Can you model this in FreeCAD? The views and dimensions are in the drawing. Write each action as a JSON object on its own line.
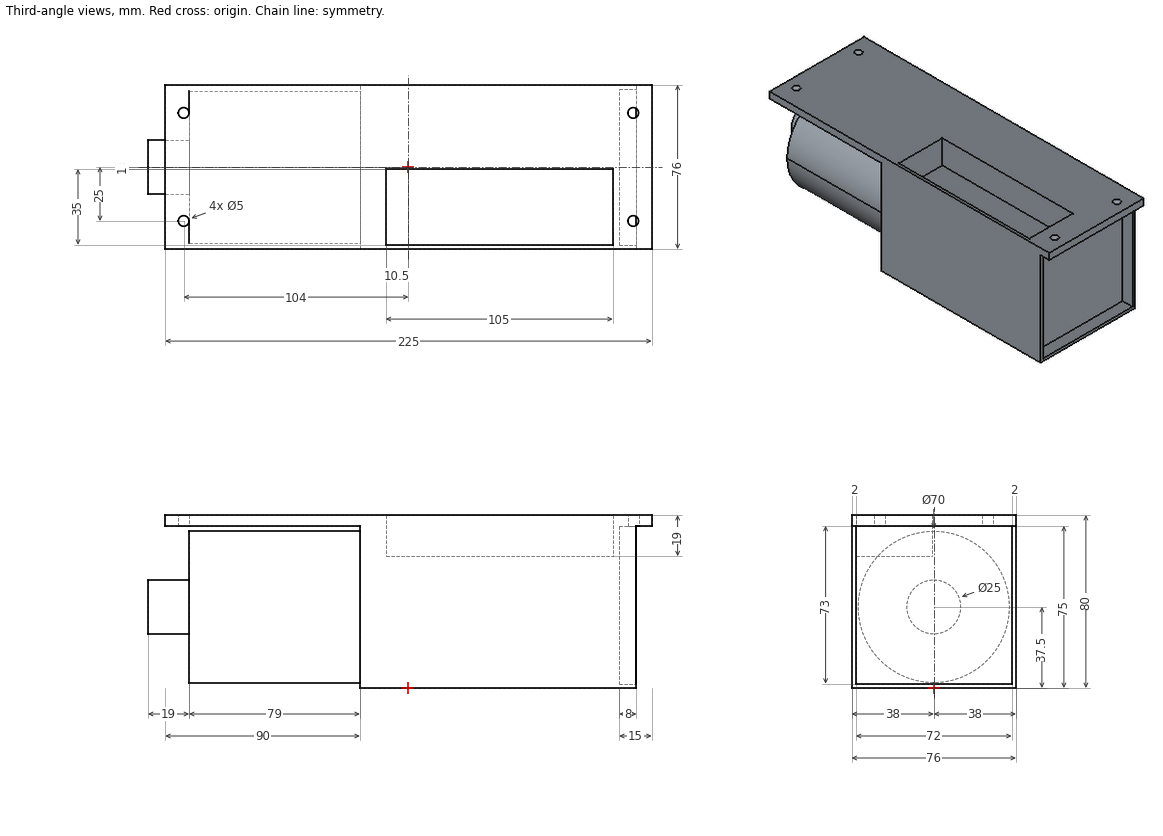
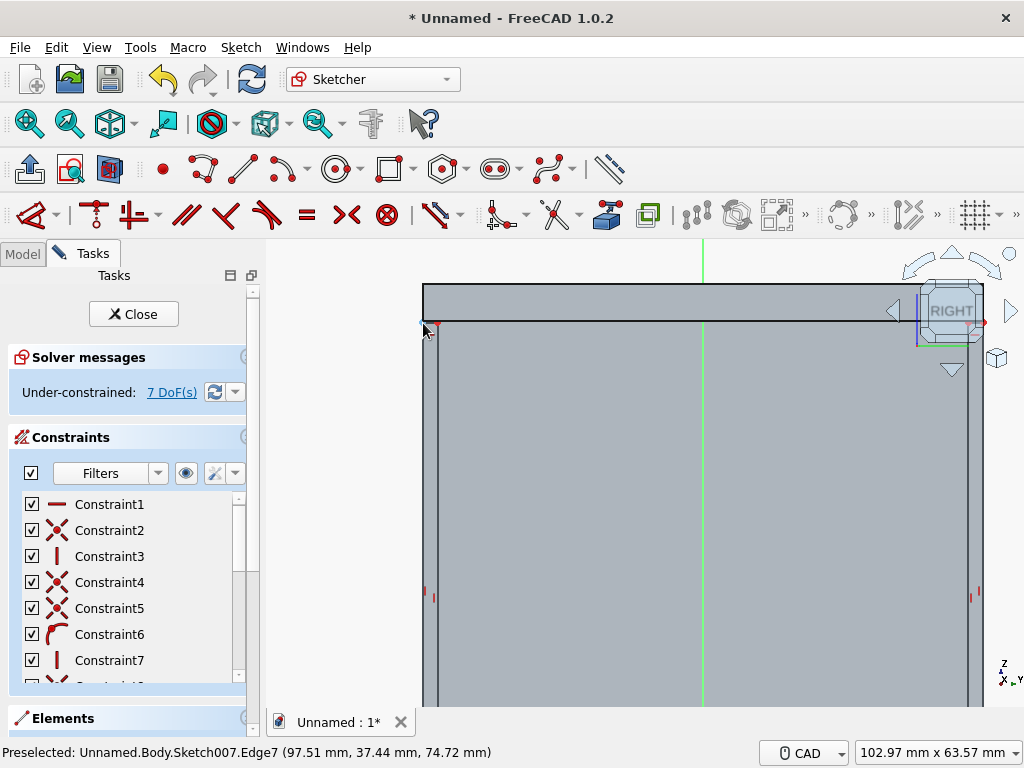
{"action": "left_click", "coordinate": [423, 323]}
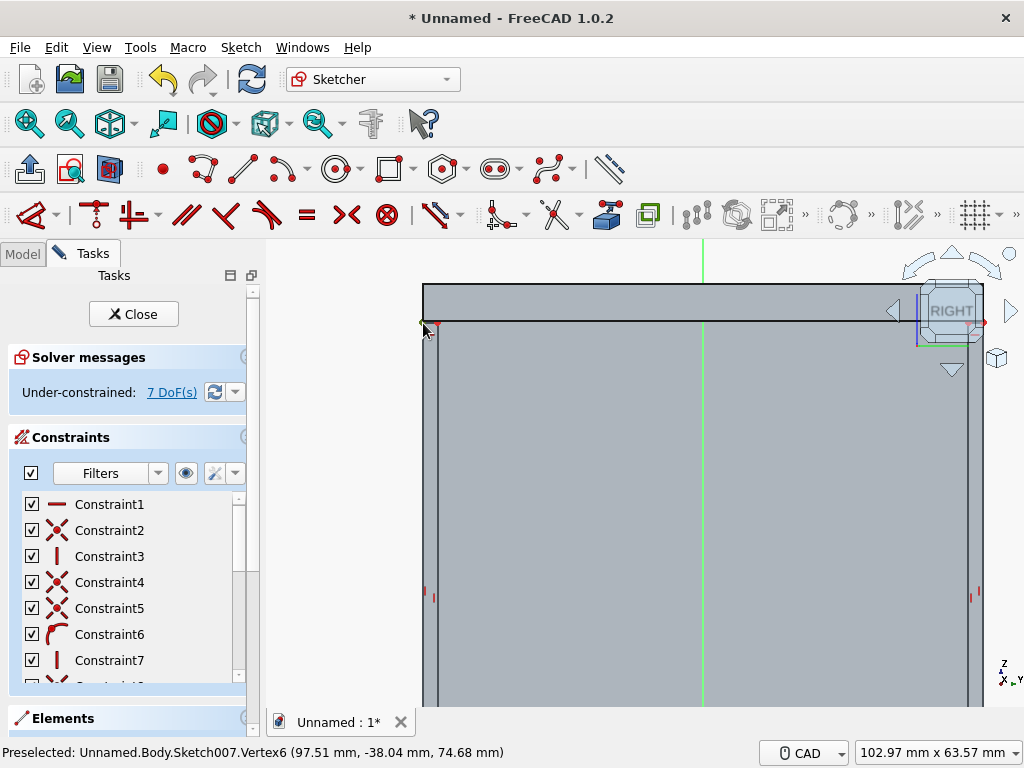
{"action": "scroll", "coordinate": [423, 323], "scroll_direction": "down", "scroll_amount": 3}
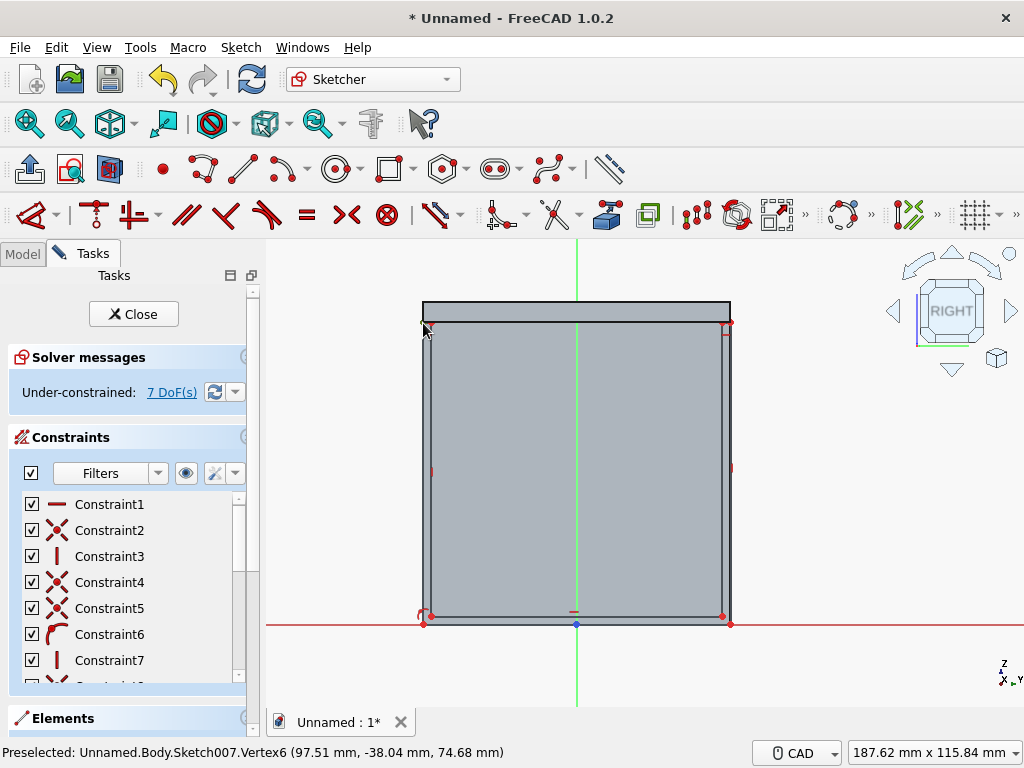
{"action": "scroll", "coordinate": [731, 323], "scroll_direction": "up", "scroll_amount": 2}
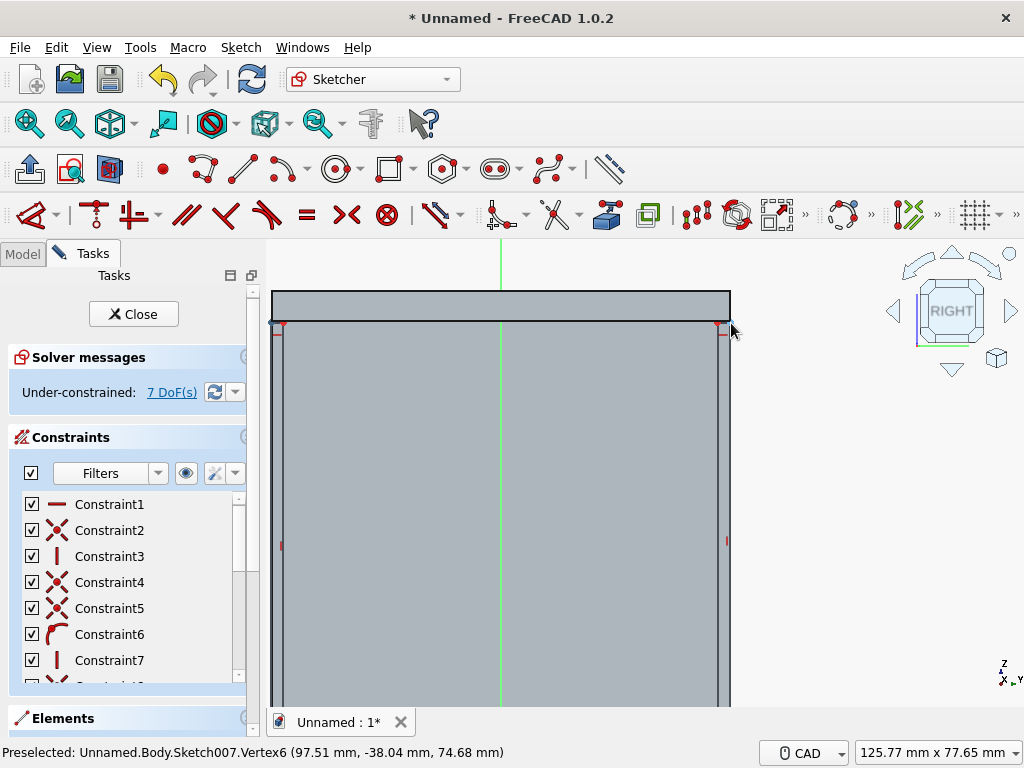
{"action": "left_click", "coordinate": [730, 323]}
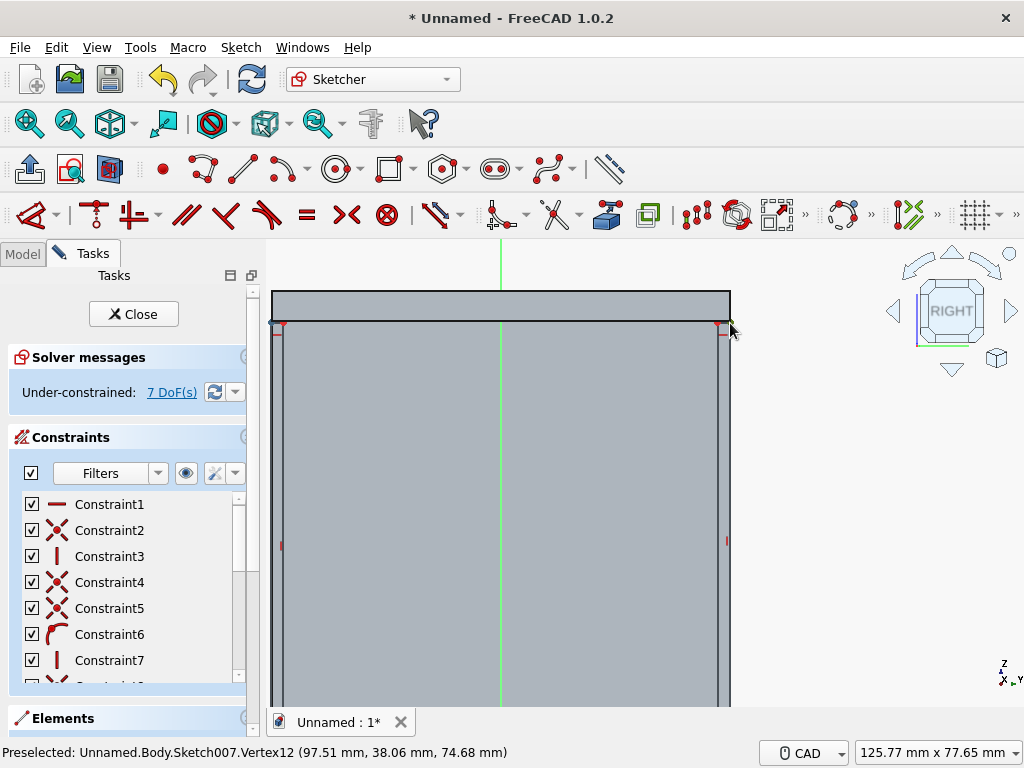
{"action": "left_click", "coordinate": [501, 650]}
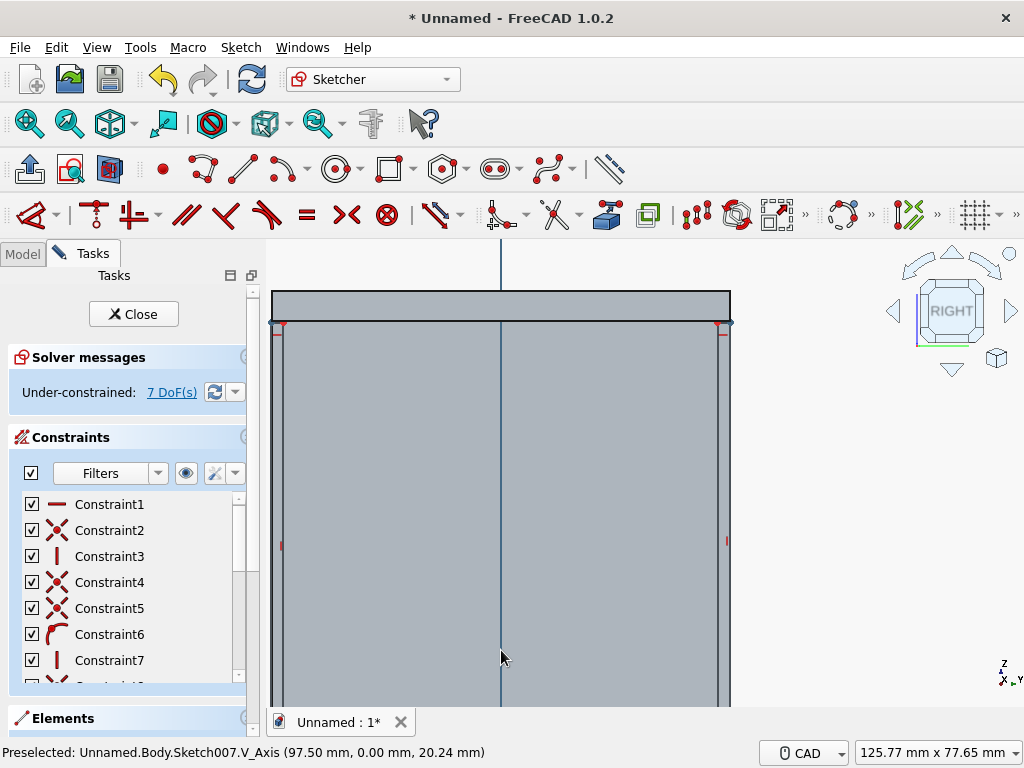
{"action": "key", "text": "s"}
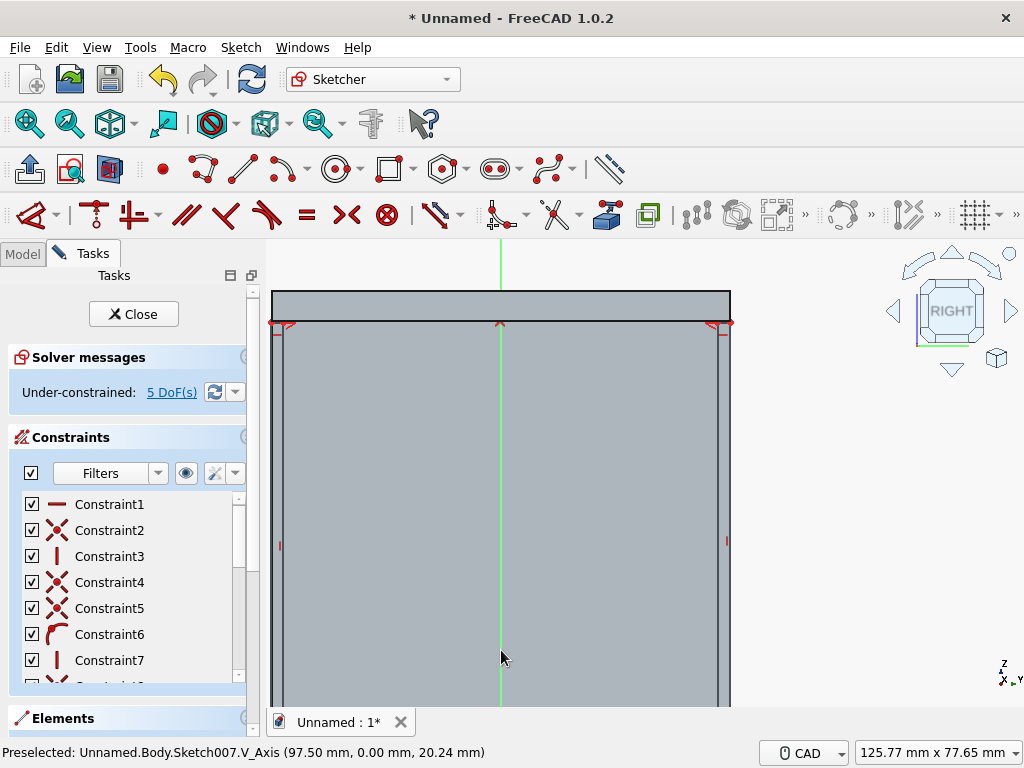
{"action": "left_click", "coordinate": [32, 216]}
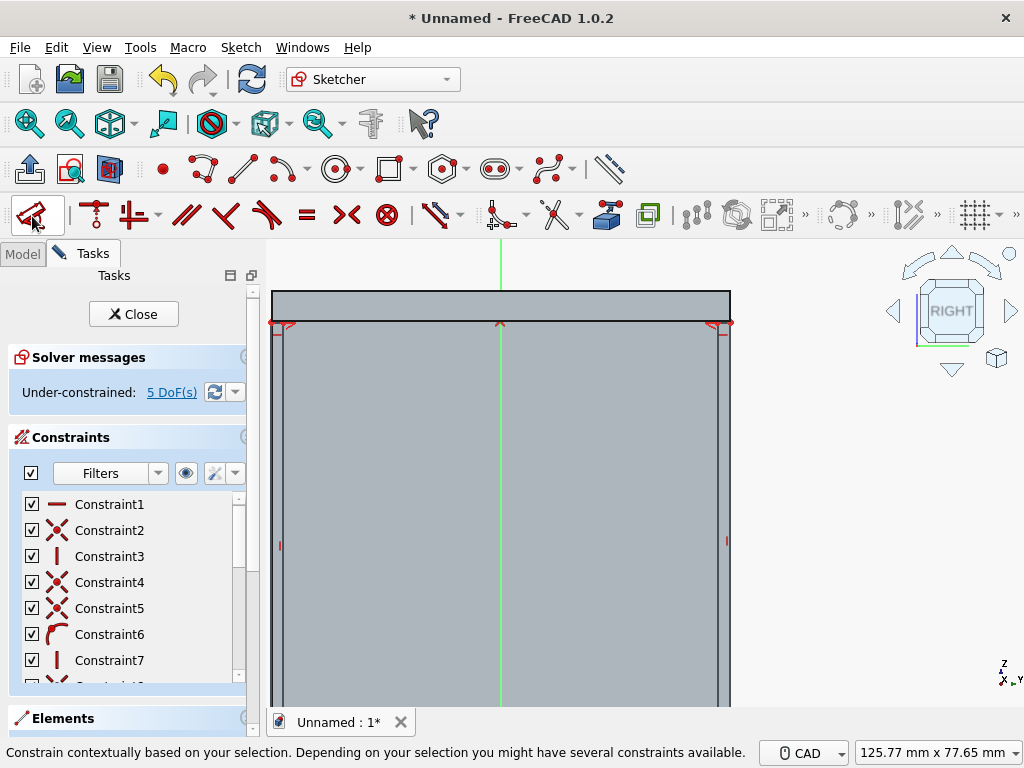
{"action": "scroll", "coordinate": [731, 323], "scroll_direction": "down", "scroll_amount": 2}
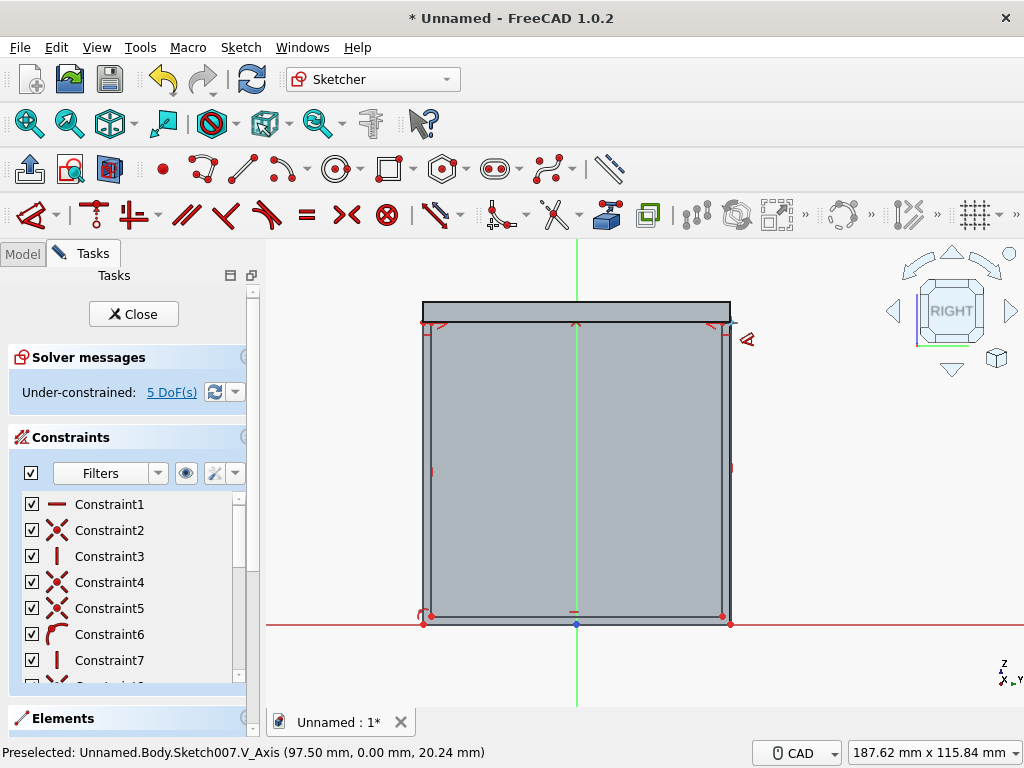
{"action": "scroll", "coordinate": [427, 323], "scroll_direction": "up", "scroll_amount": 8}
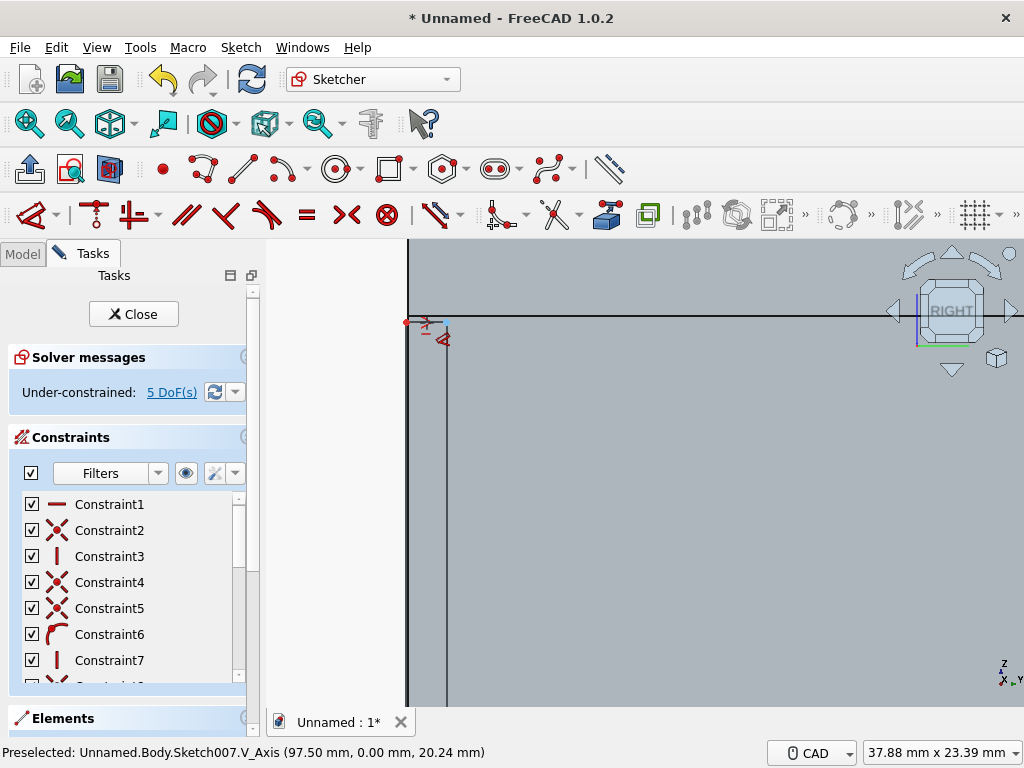
{"action": "left_click", "coordinate": [426, 322]}
{"action": "left_click", "coordinate": [426, 288]}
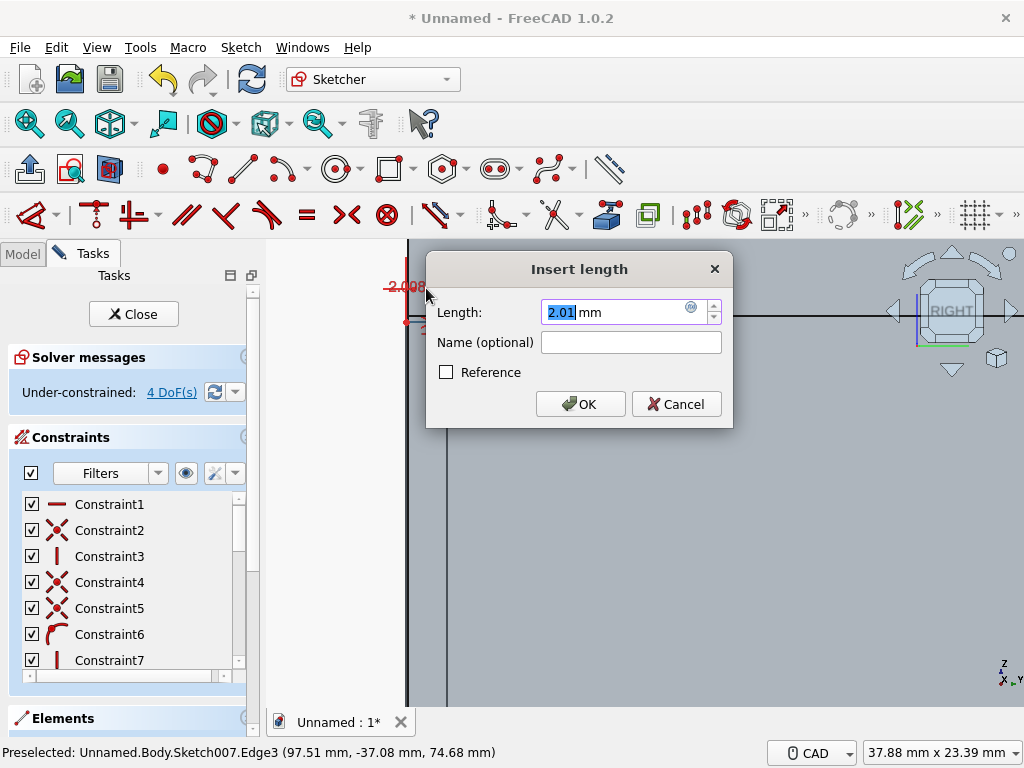
{"action": "type", "text": "2"}
{"action": "key", "text": "Return"}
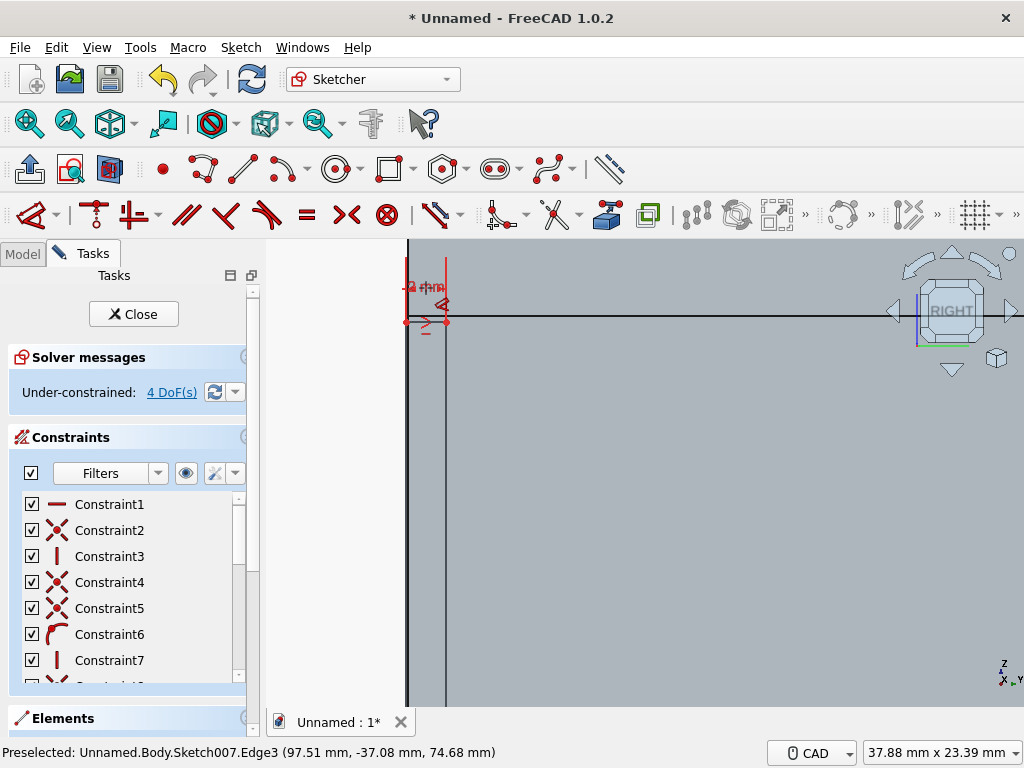
{"action": "scroll", "coordinate": [427, 323], "scroll_direction": "down", "scroll_amount": 8}